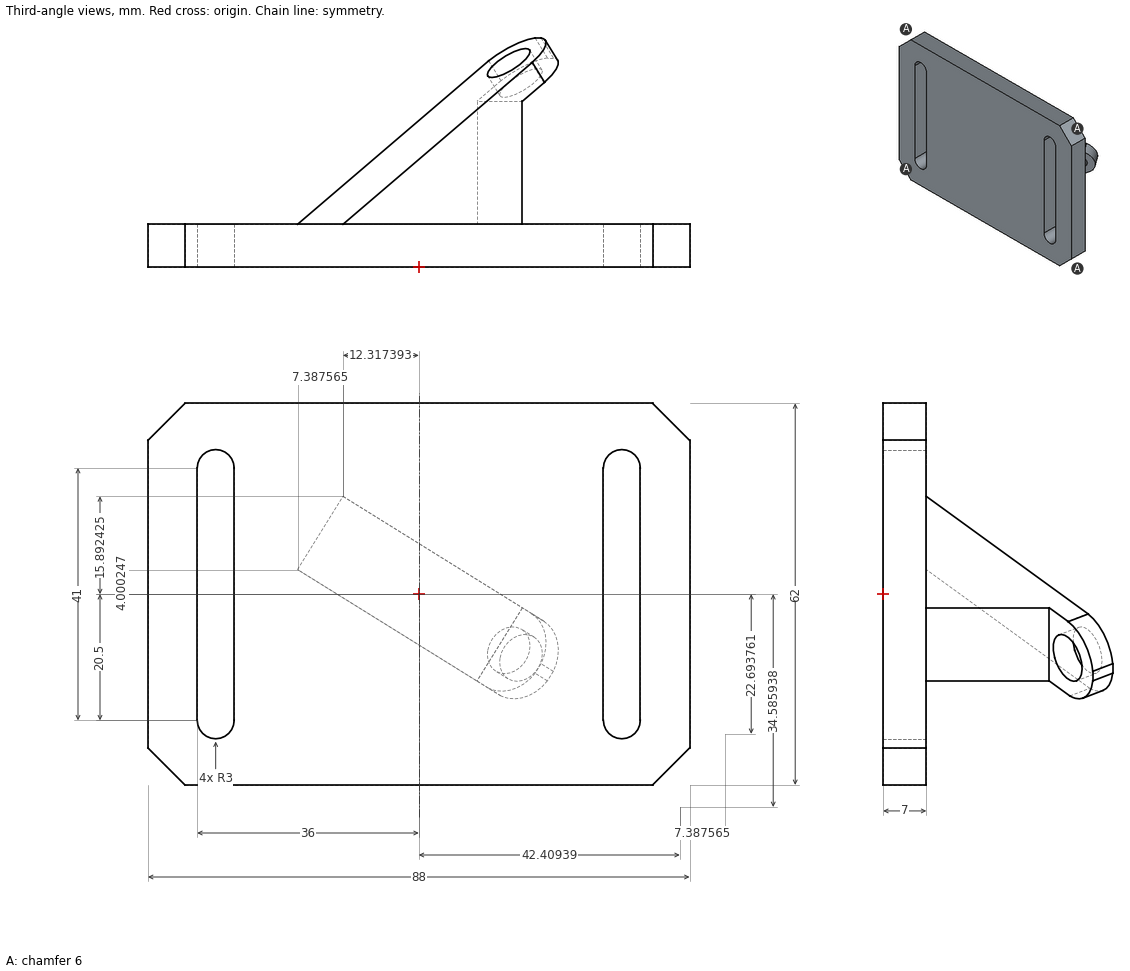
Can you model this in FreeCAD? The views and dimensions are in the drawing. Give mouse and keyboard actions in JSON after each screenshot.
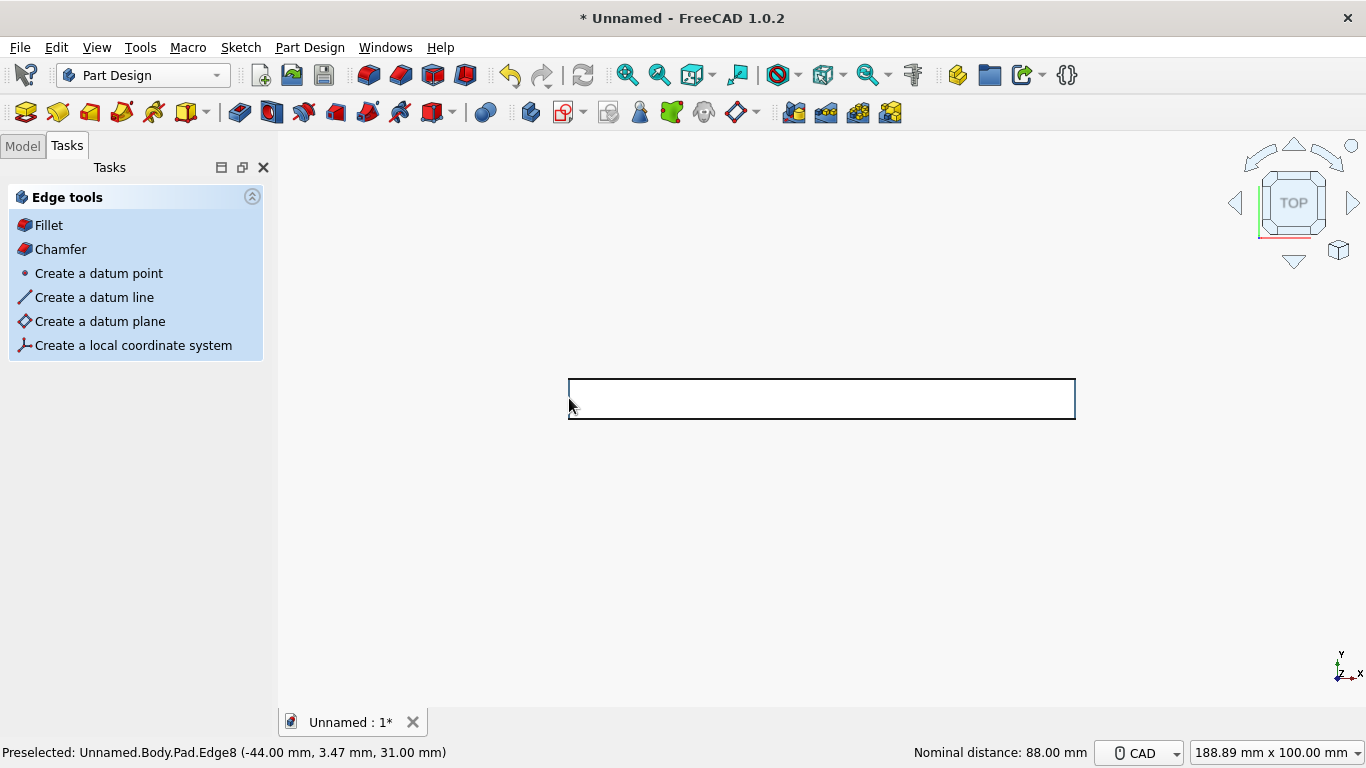
{"action": "key", "text": "1"}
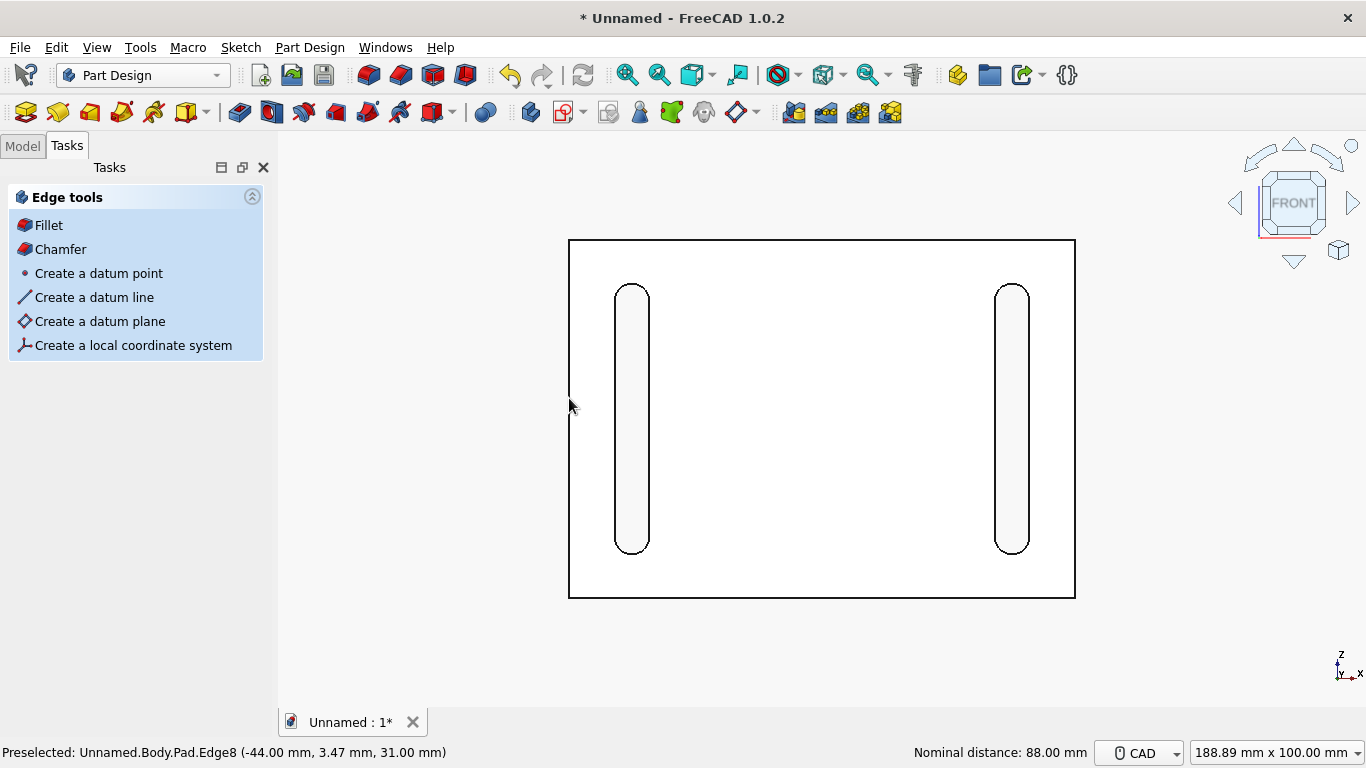
{"action": "key", "text": "3"}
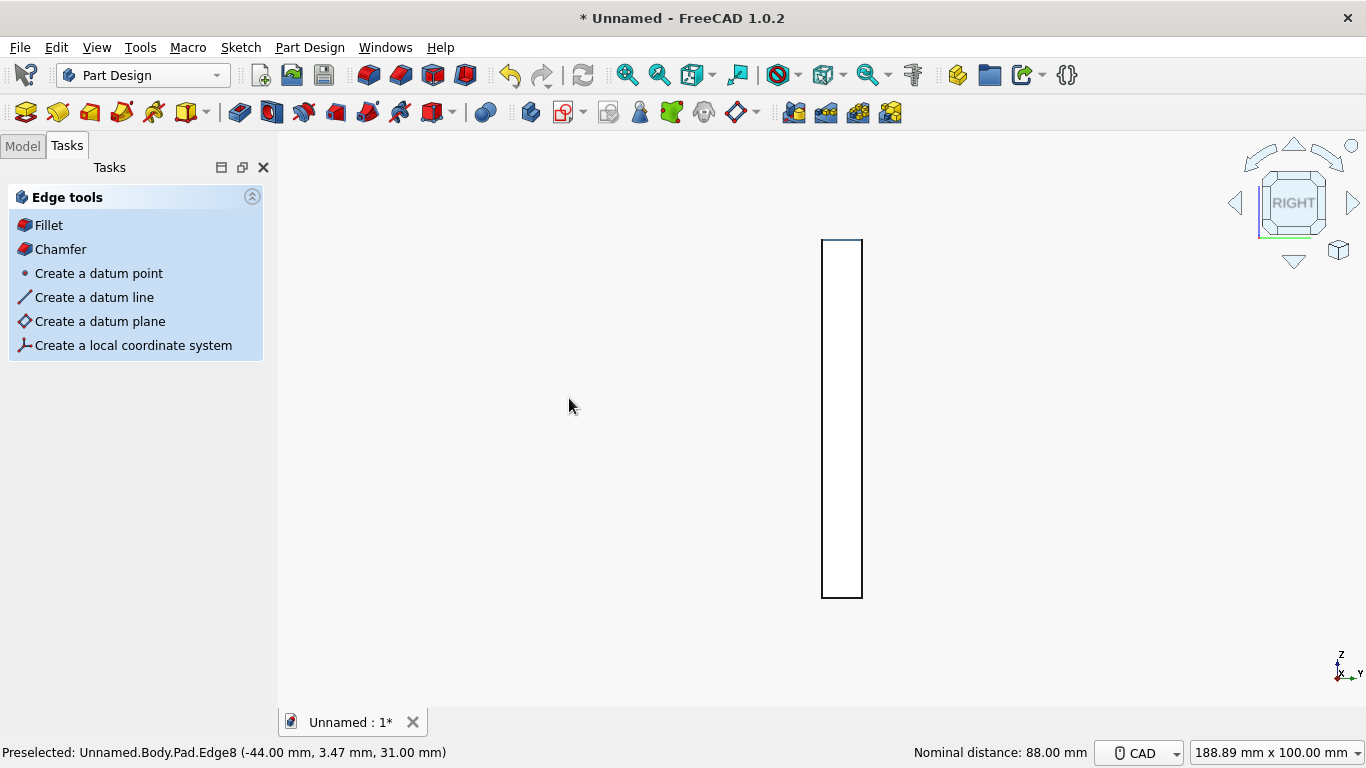
{"action": "left_click", "coordinate": [842, 597], "text": "ctrl"}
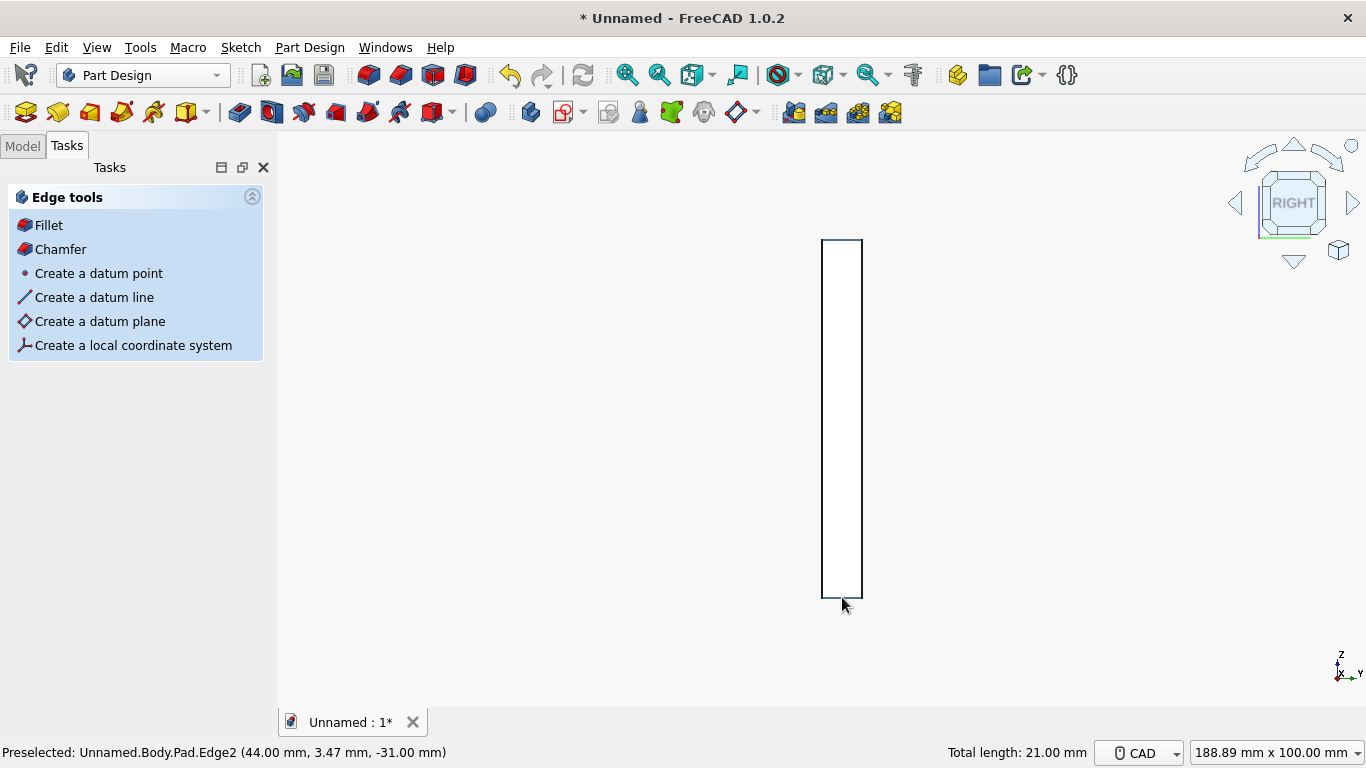
{"action": "key", "text": "5"}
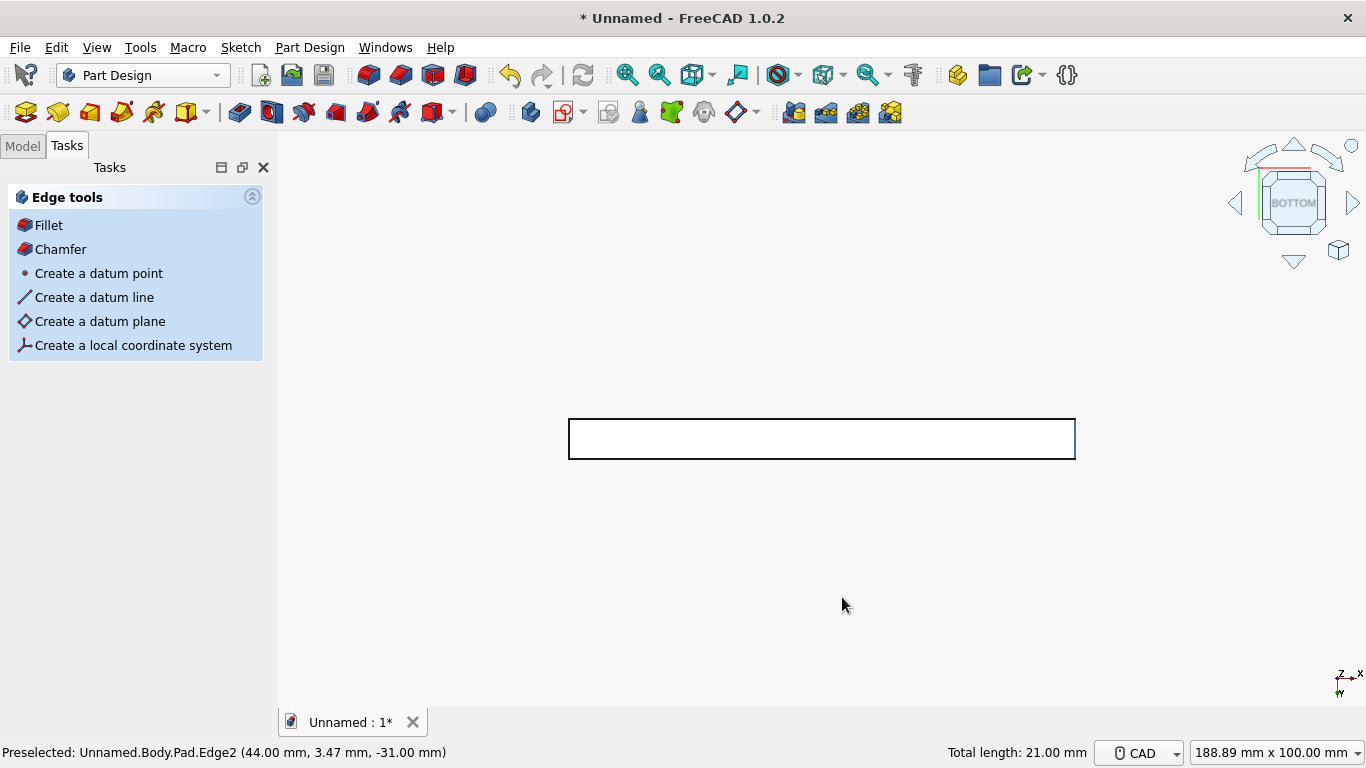
{"action": "left_click", "coordinate": [569, 438], "text": "ctrl"}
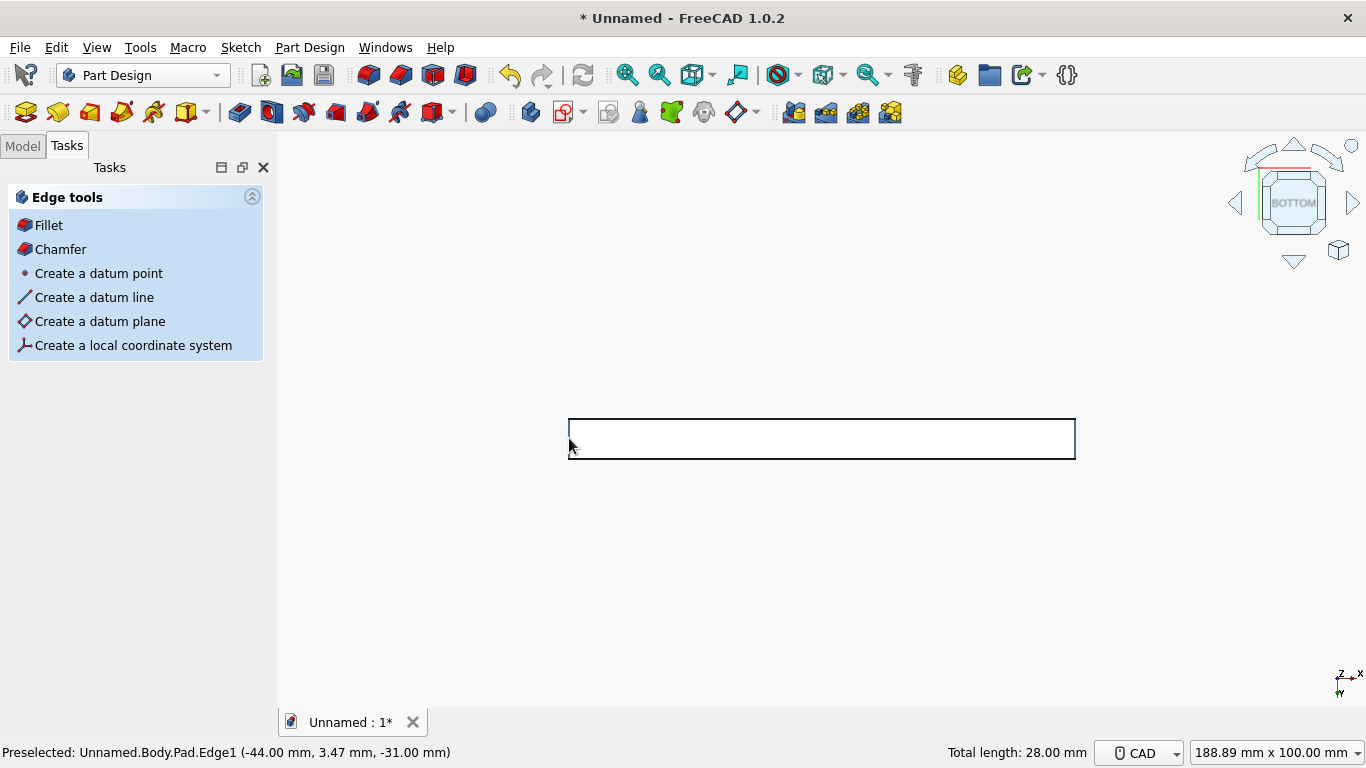
{"action": "left_click", "coordinate": [402, 76]}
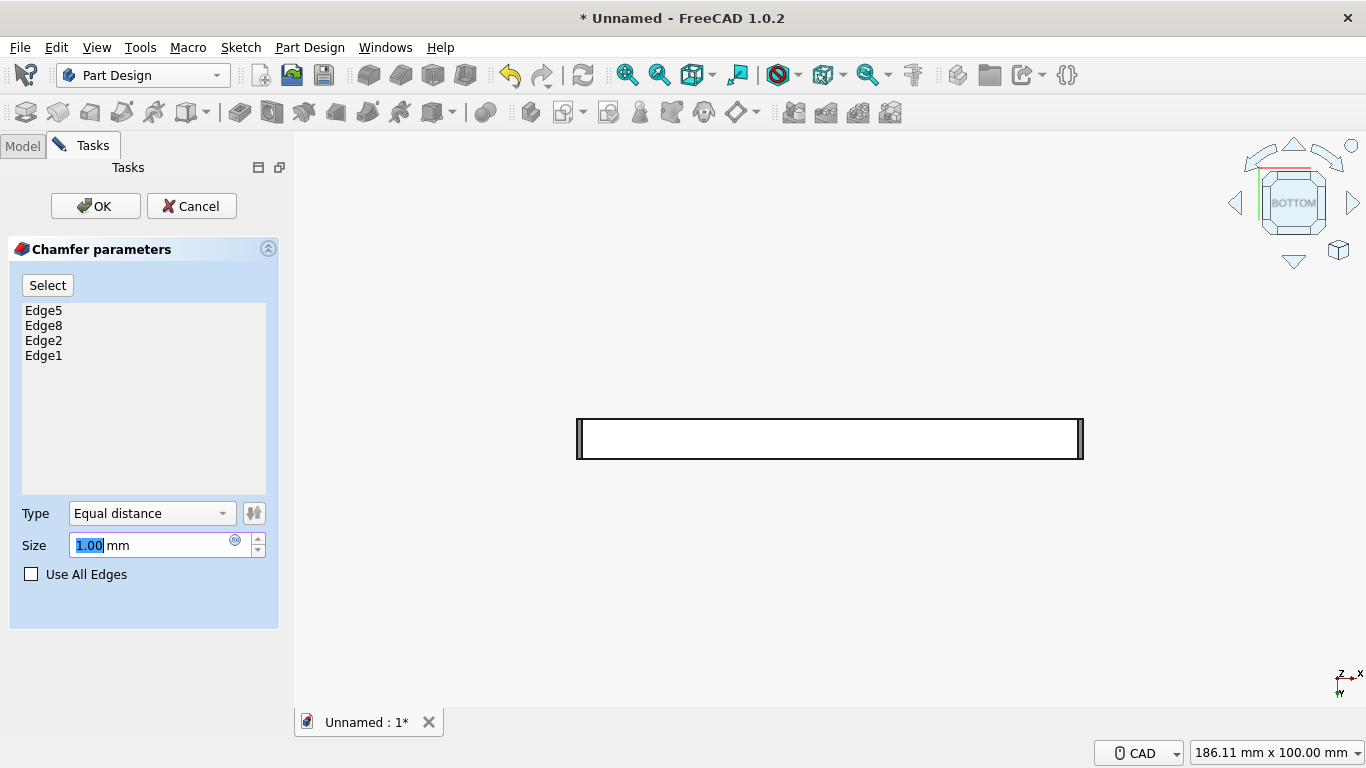
{"action": "type", "text": "6"}
{"action": "key", "text": "Tab"}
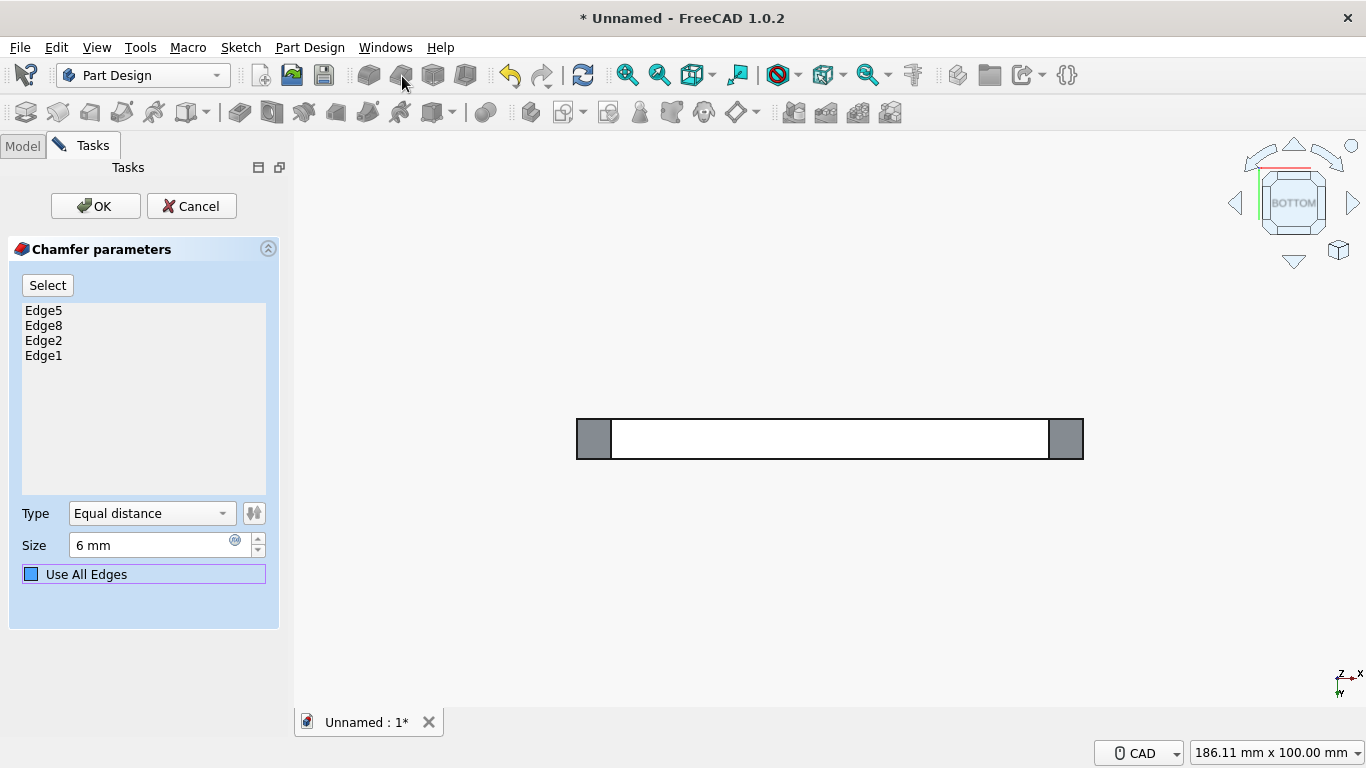
{"action": "left_click", "coordinate": [96, 206]}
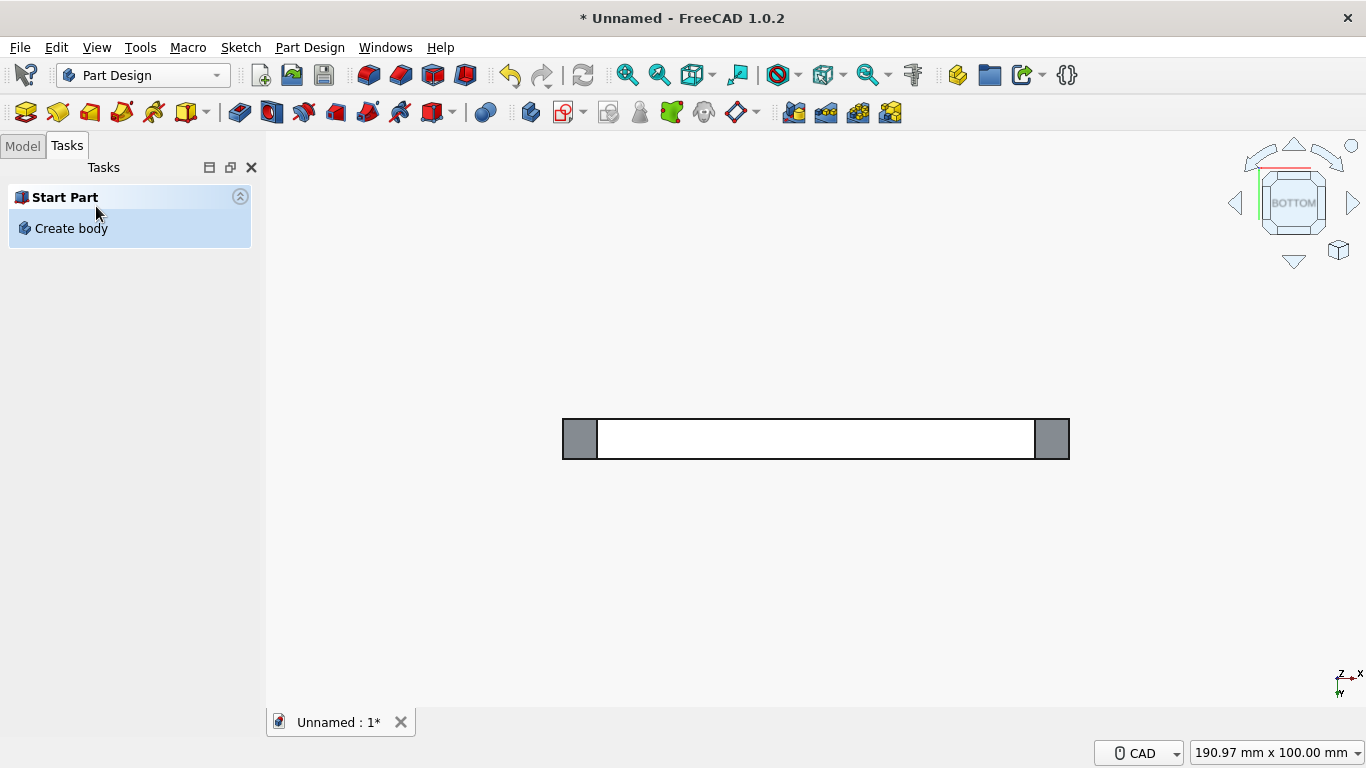
{"action": "key", "text": "4"}